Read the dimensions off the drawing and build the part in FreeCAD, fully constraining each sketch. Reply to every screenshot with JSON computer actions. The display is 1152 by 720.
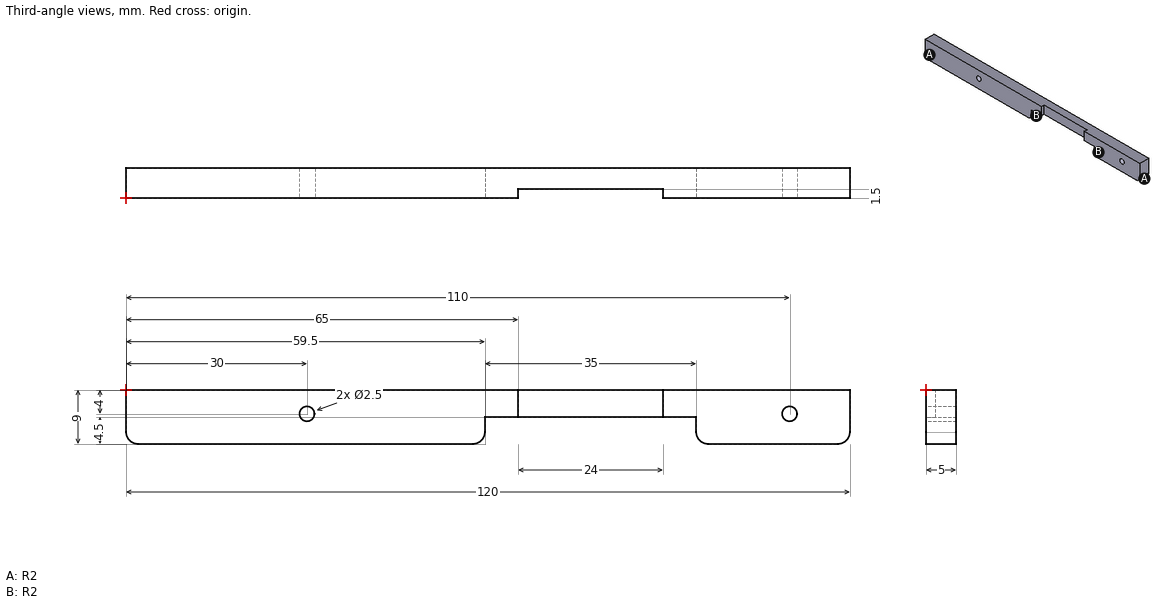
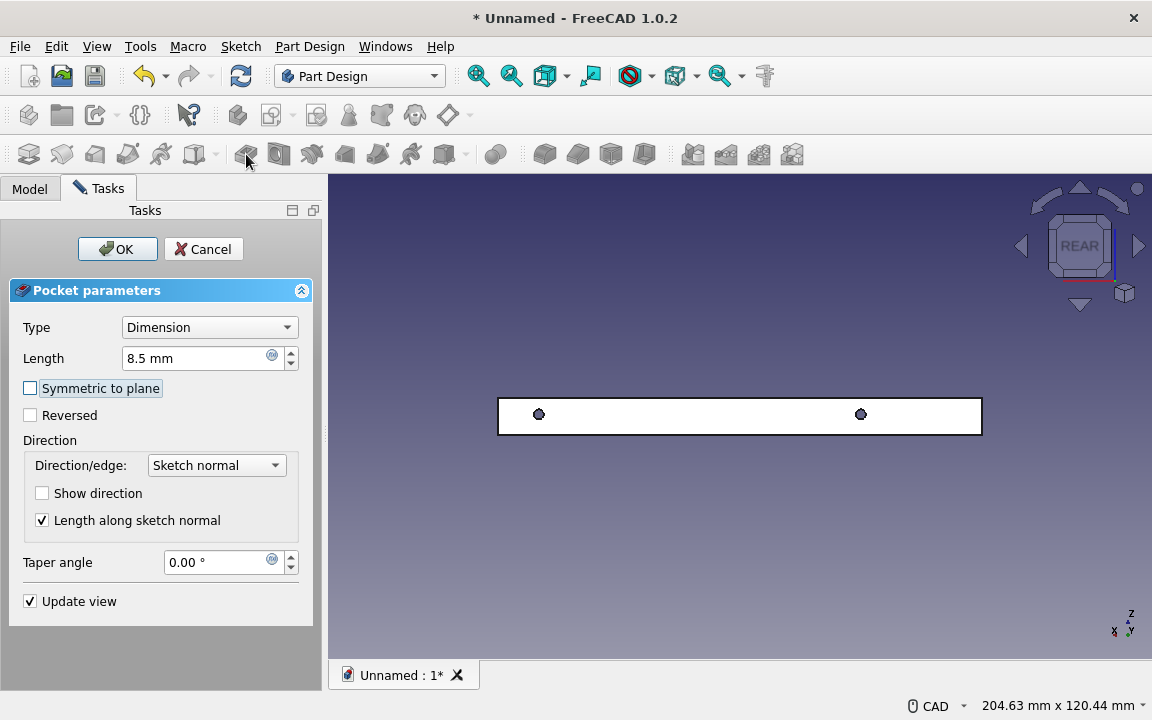
{"action": "left_click", "coordinate": [118, 249]}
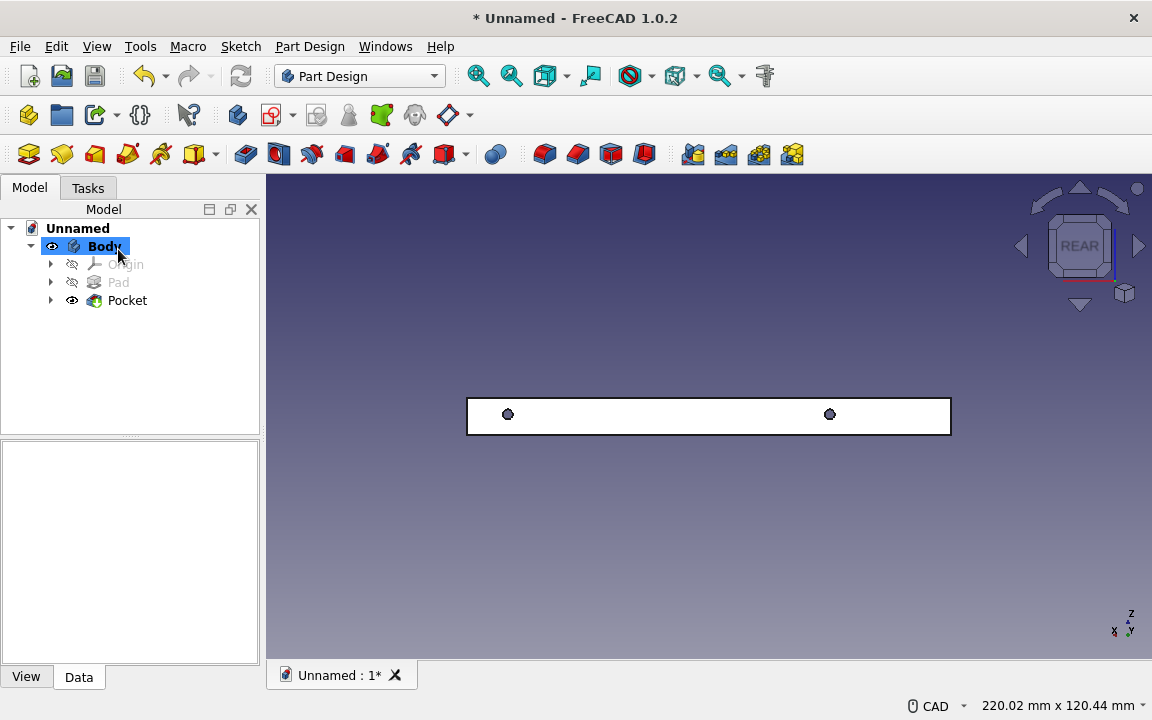
{"action": "scroll", "coordinate": [951, 434], "scroll_direction": "up", "scroll_amount": 4}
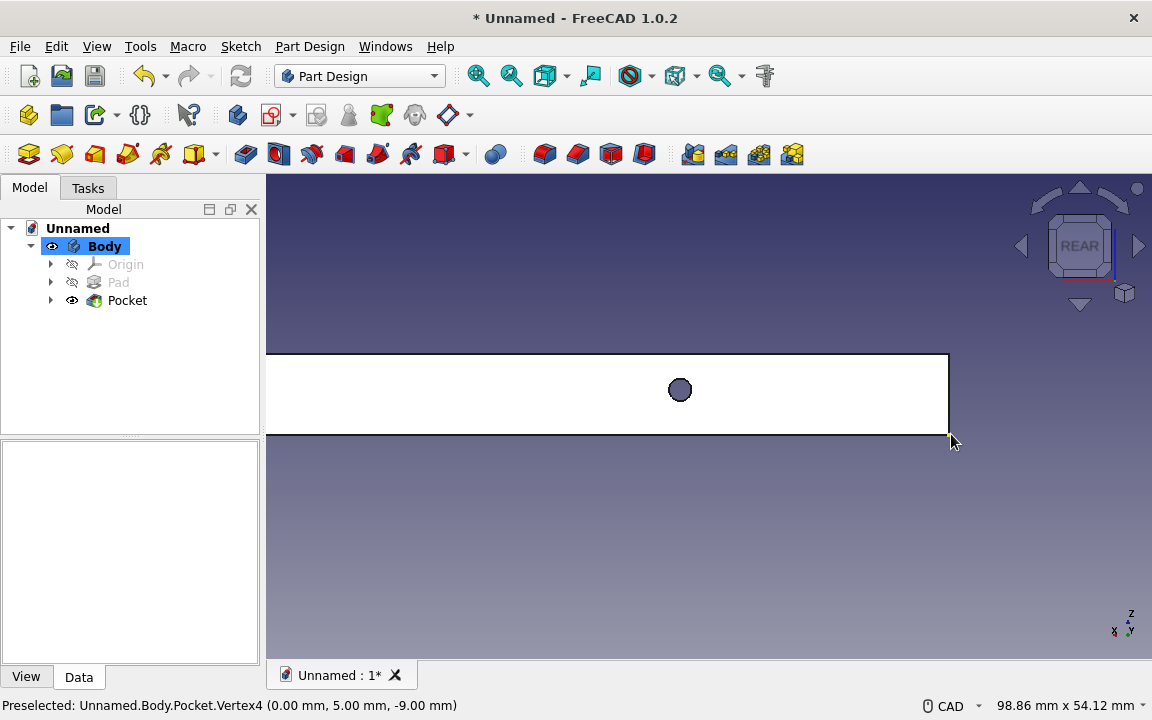
{"action": "key", "text": "v f"}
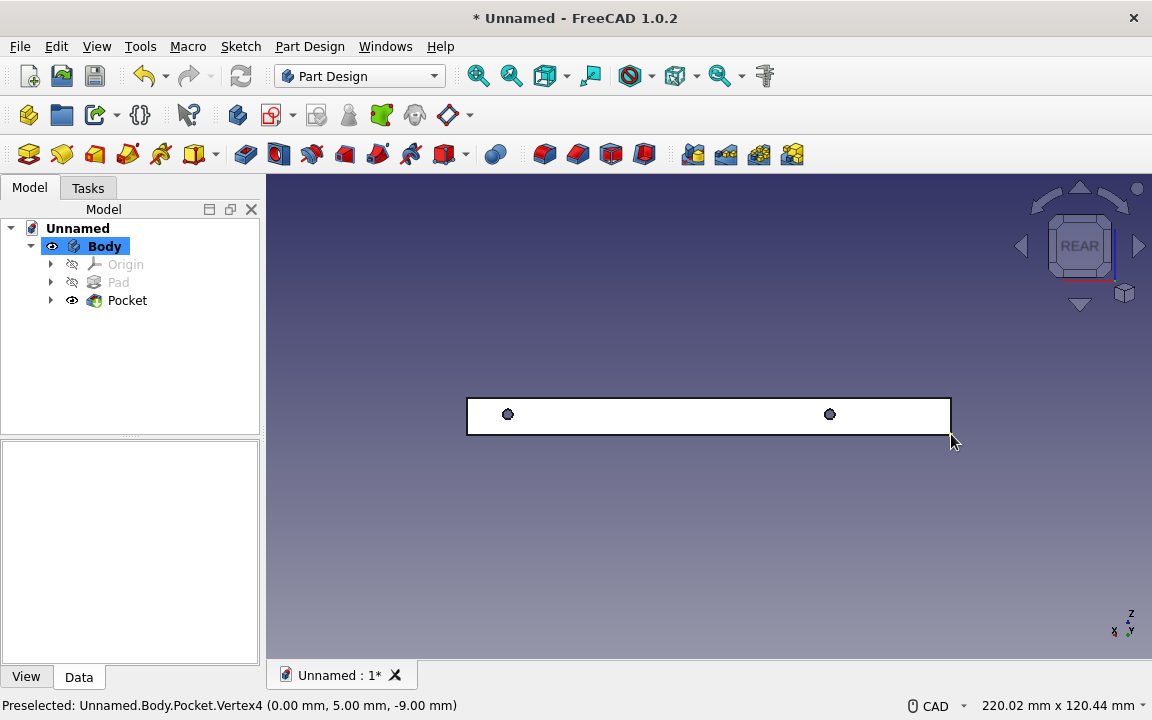
{"action": "key", "text": "0"}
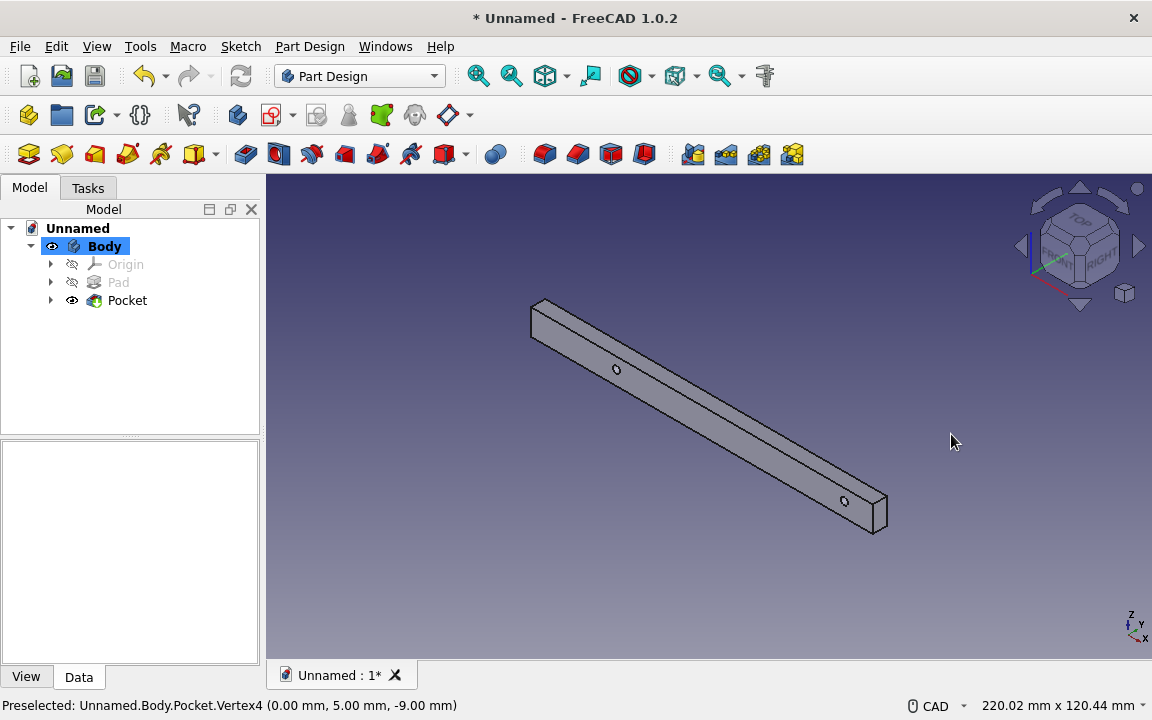
{"action": "scroll", "coordinate": [538, 332], "scroll_direction": "up", "scroll_amount": 4}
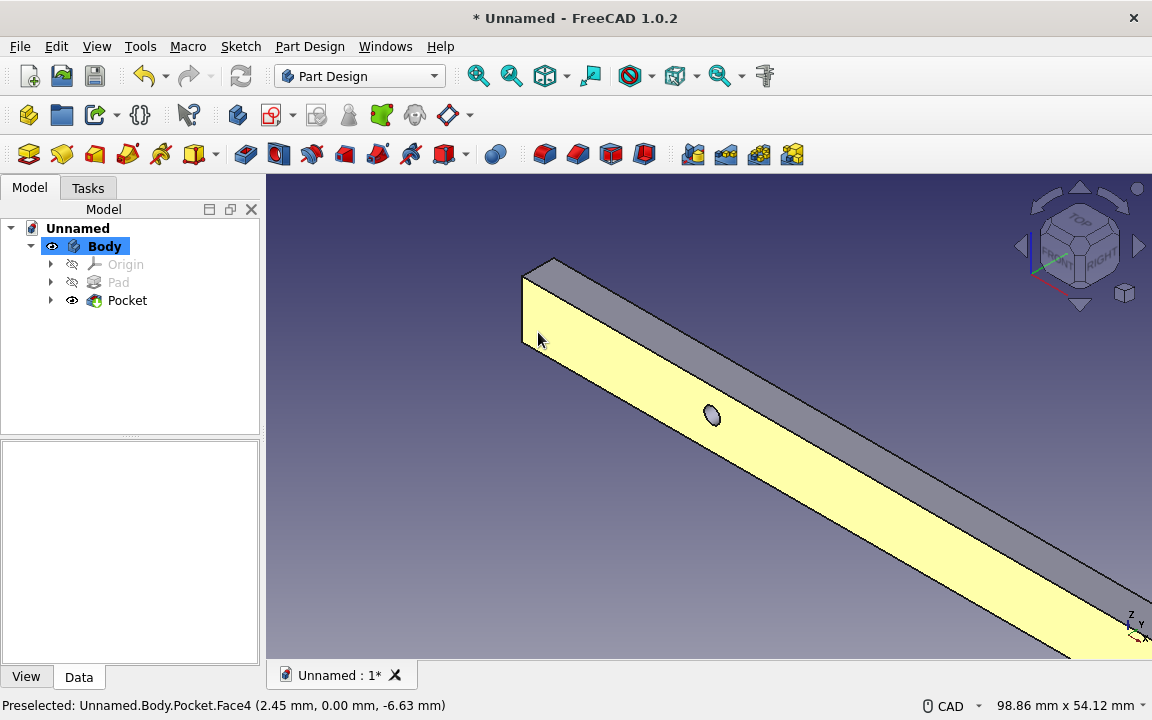
{"action": "key", "text": "v f"}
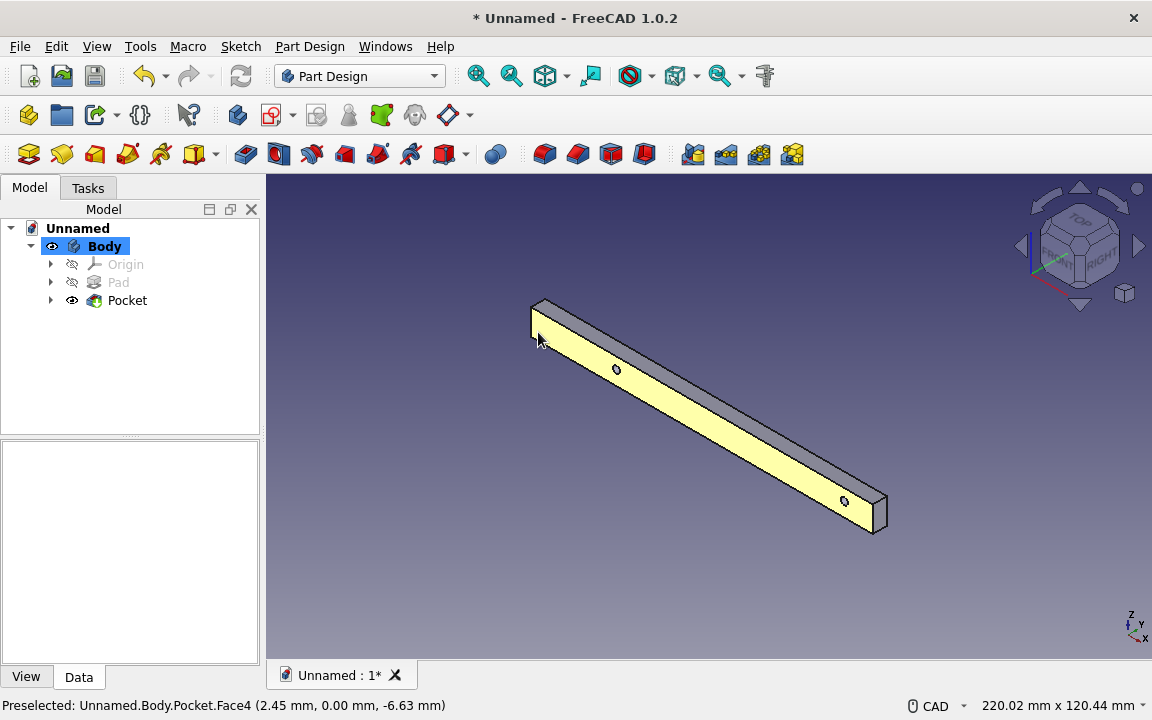
{"action": "key", "text": "2"}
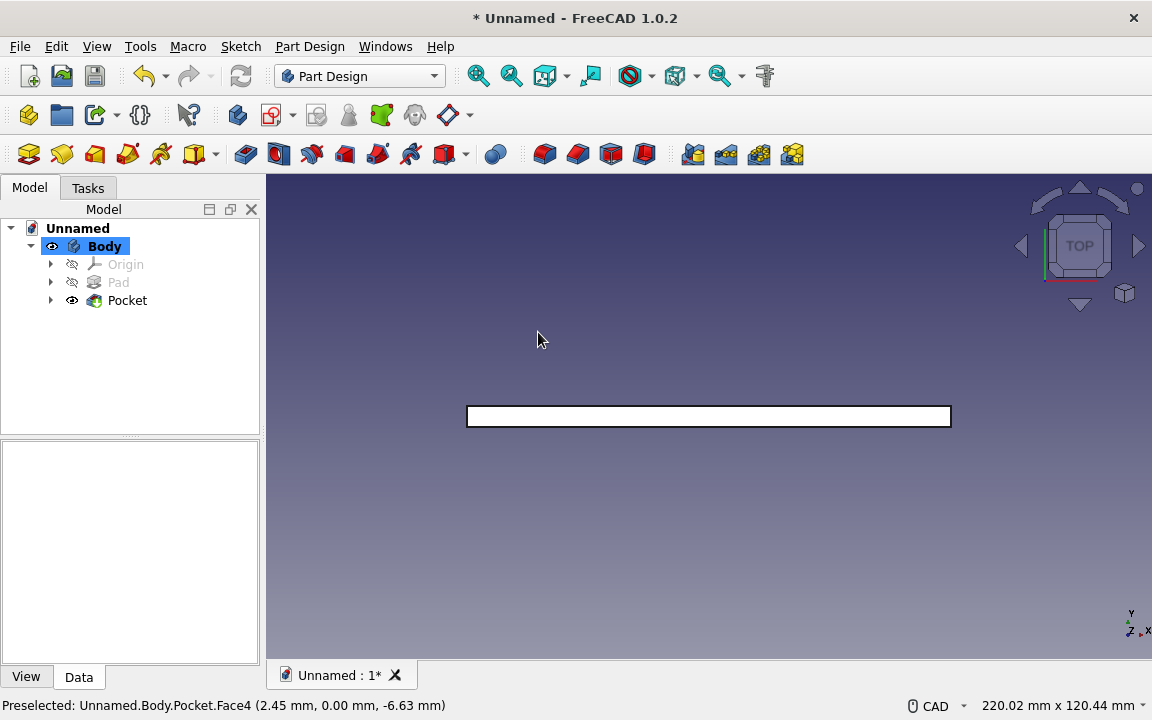
{"action": "scroll", "coordinate": [467, 415], "scroll_direction": "up", "scroll_amount": 4}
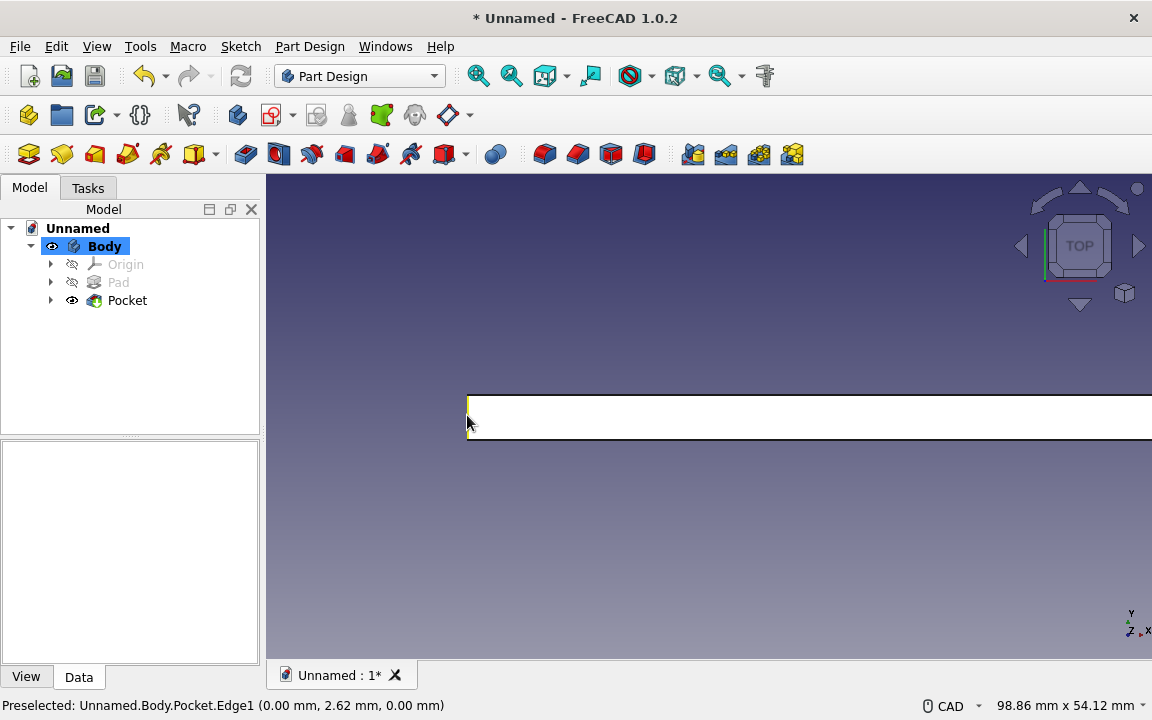
{"action": "left_click", "coordinate": [479, 76]}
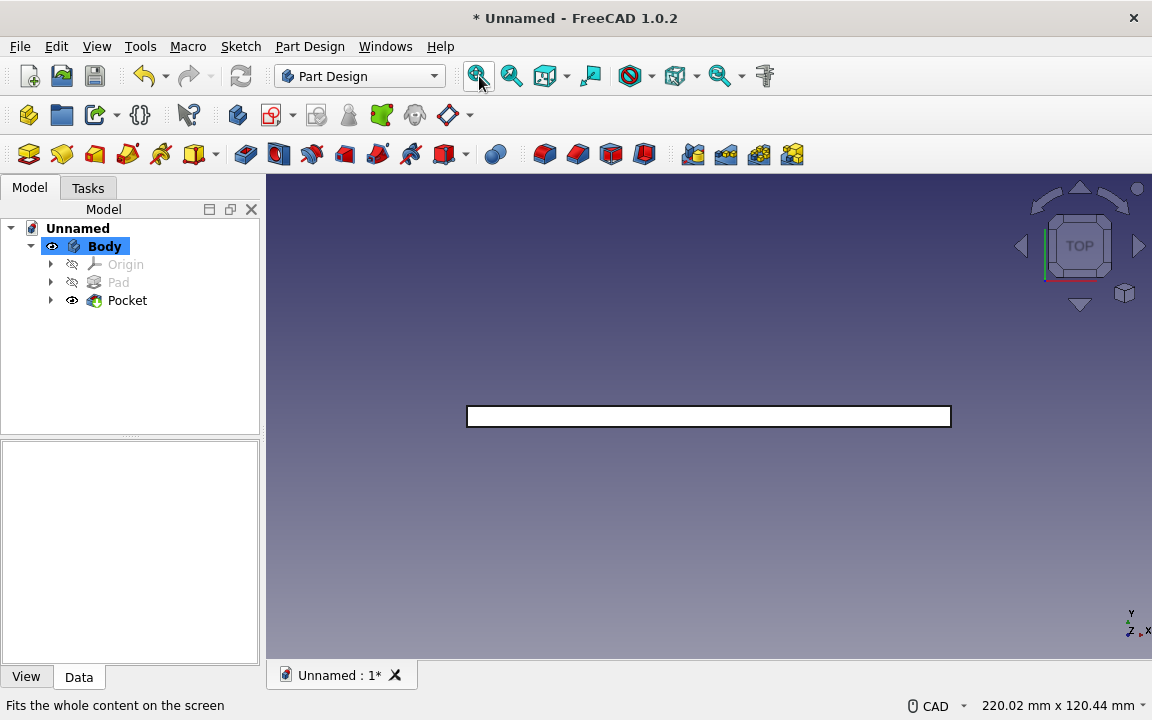
{"action": "key", "text": "1"}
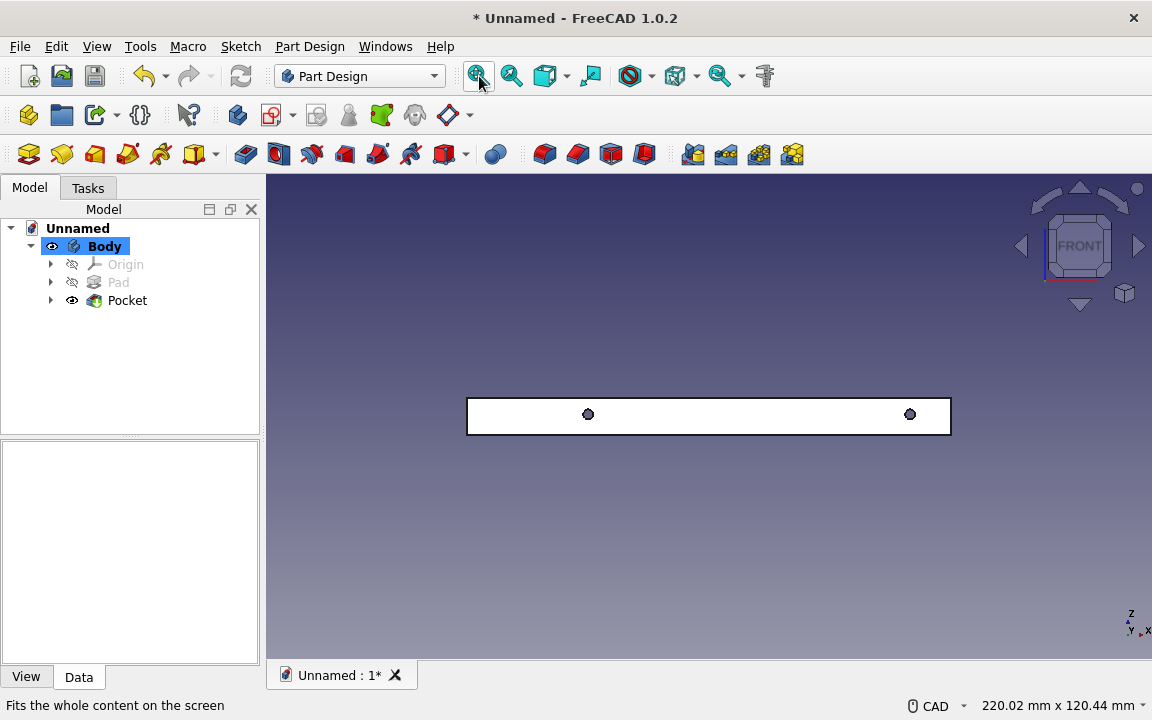
{"action": "scroll", "coordinate": [467, 434], "scroll_direction": "up", "scroll_amount": 4}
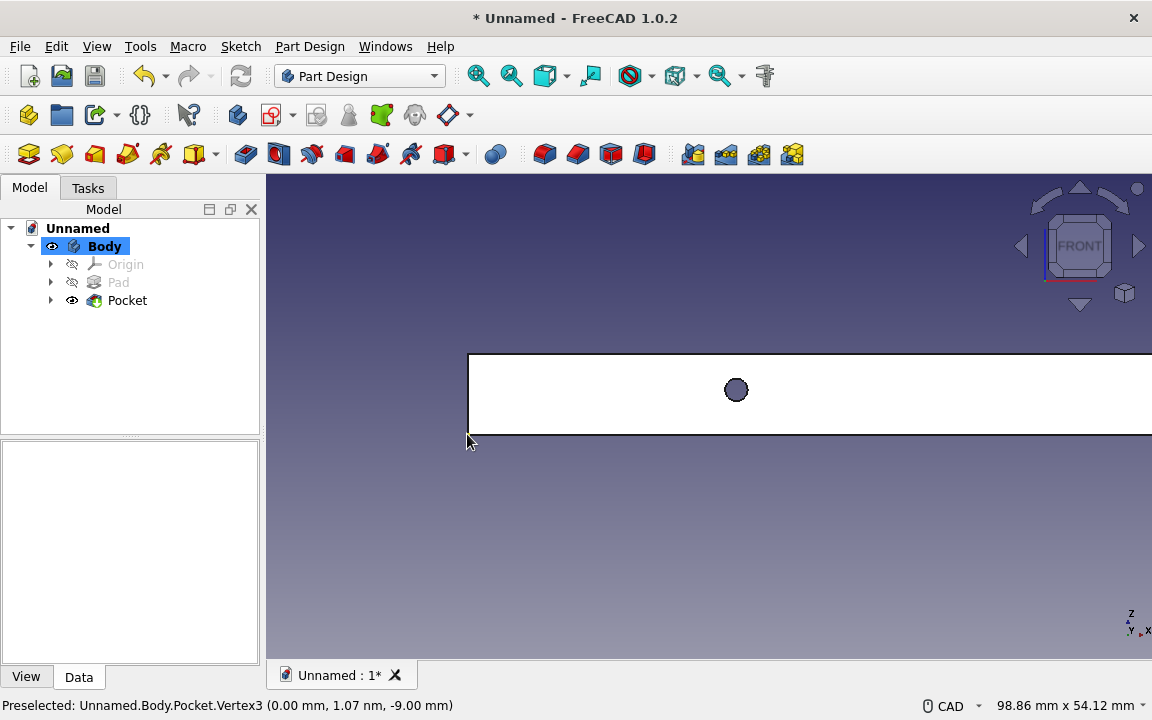
{"action": "key", "text": "v f"}